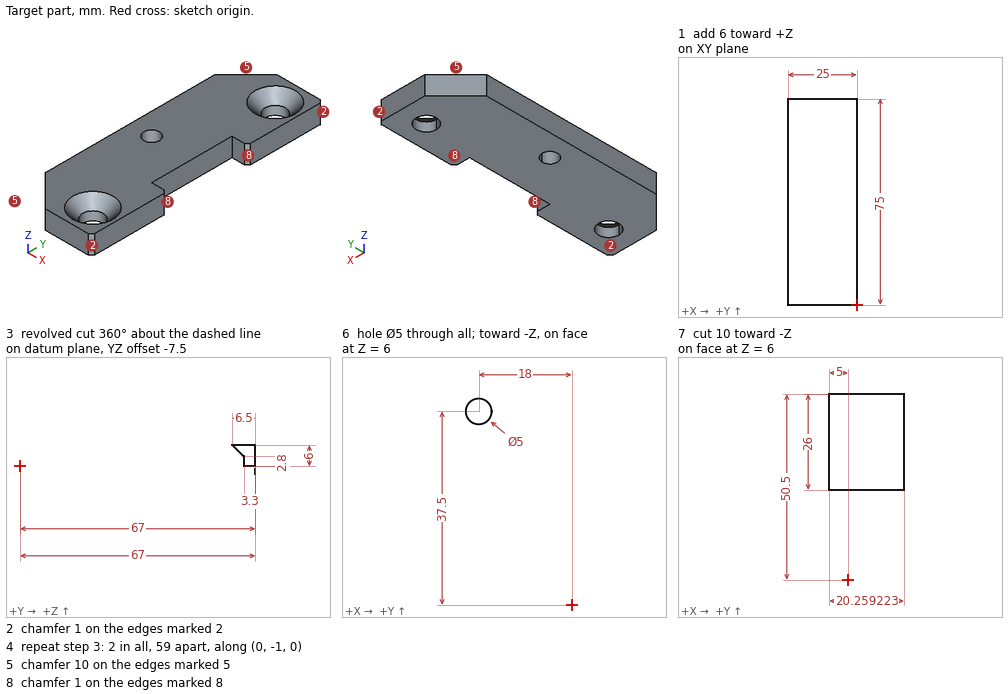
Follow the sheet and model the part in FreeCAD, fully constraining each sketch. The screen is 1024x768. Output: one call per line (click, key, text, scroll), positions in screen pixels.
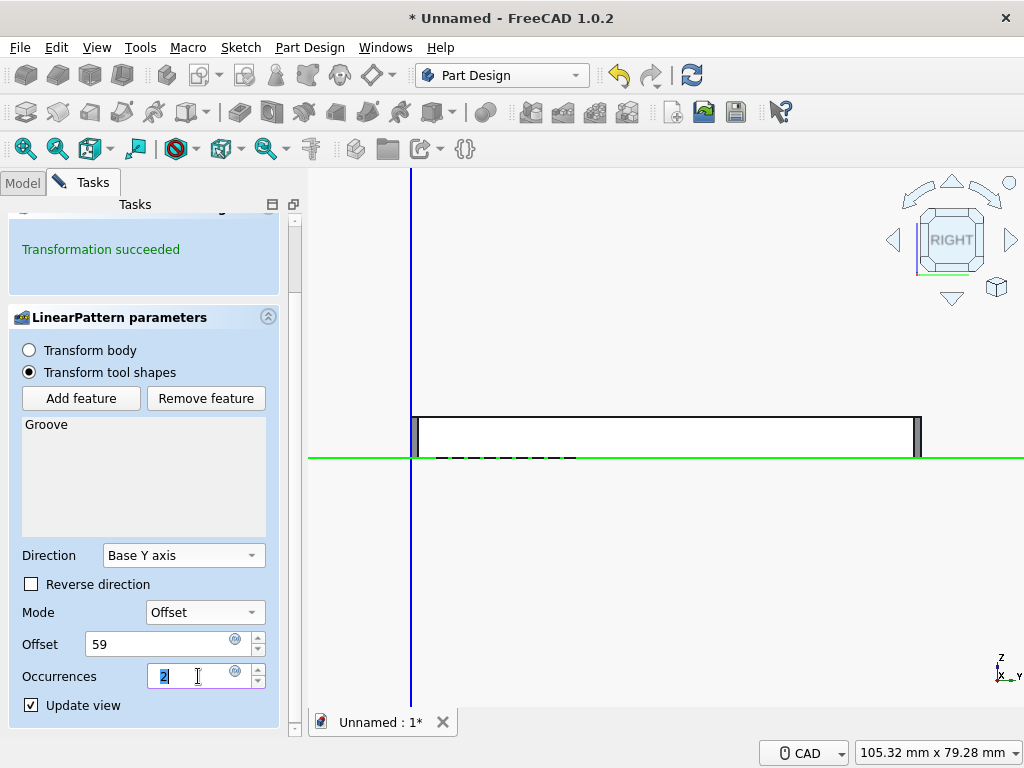
text(2)
key(Tab)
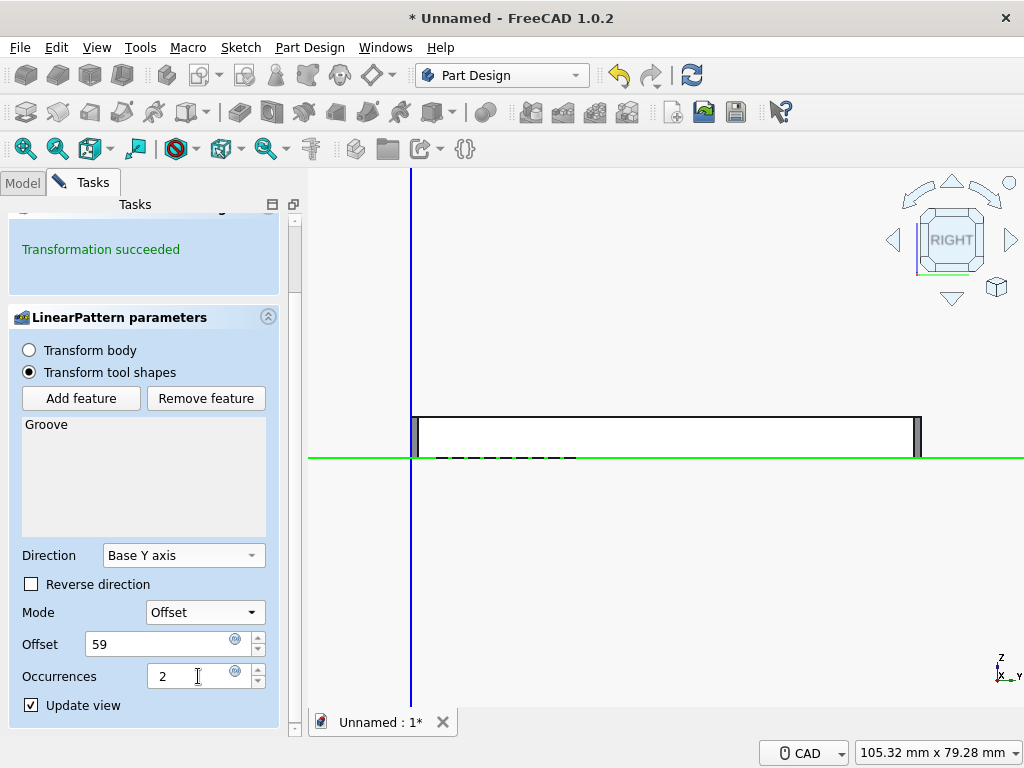
click(30, 584)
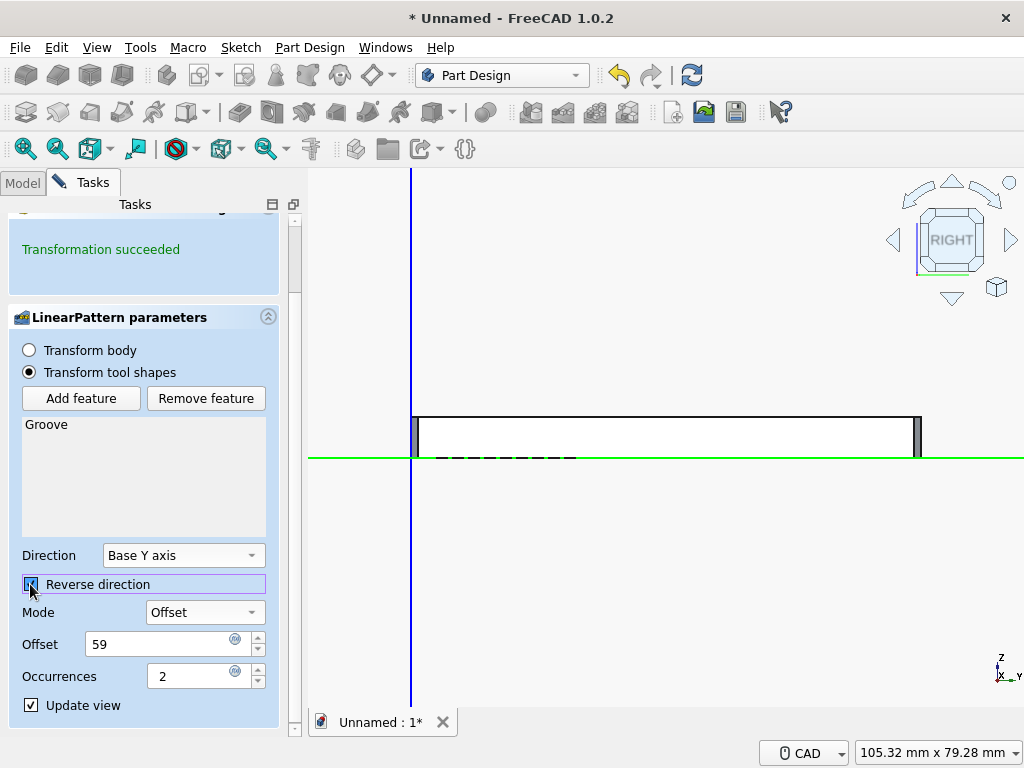
scroll(295, 475, up, 3)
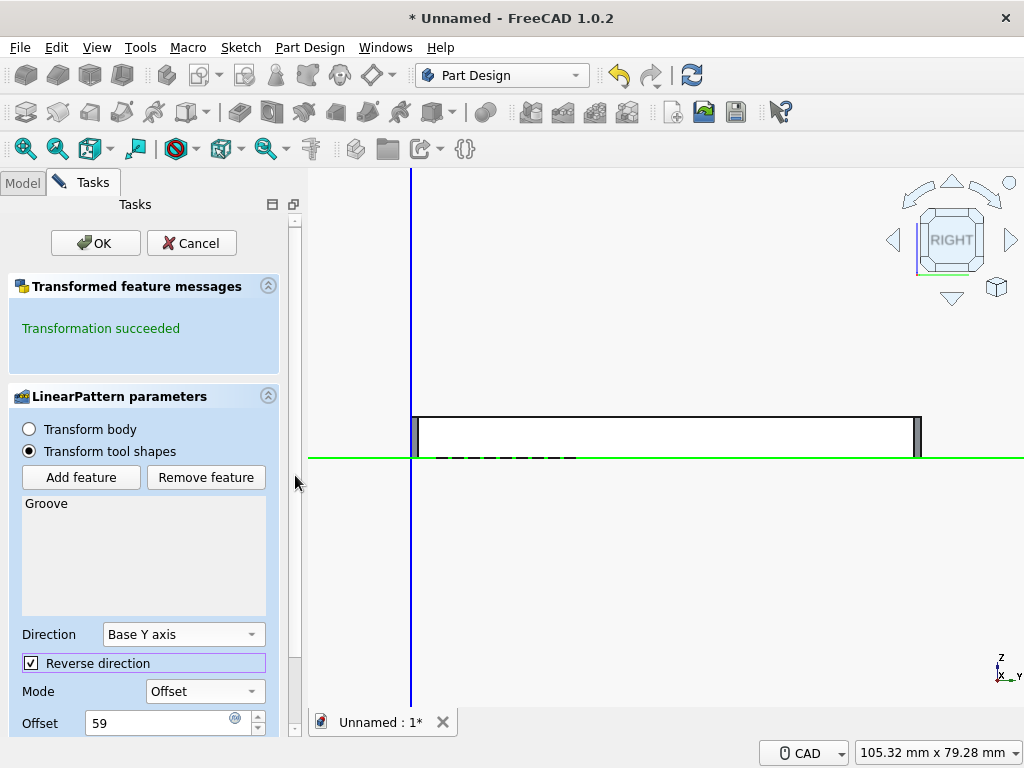
click(96, 243)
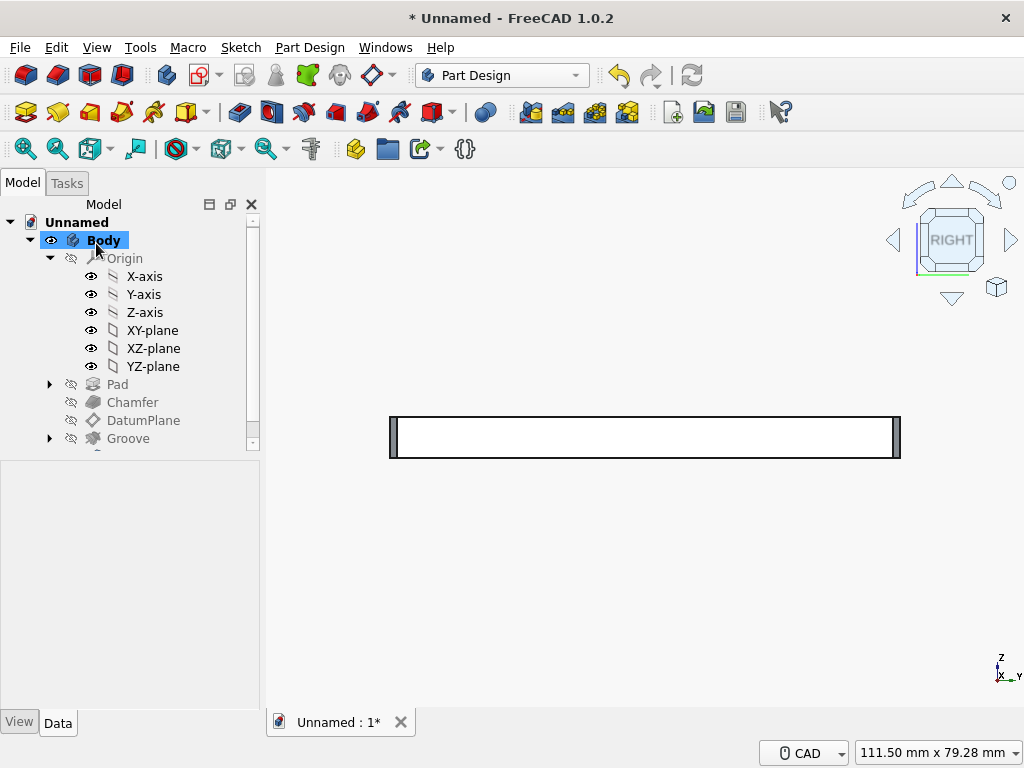
key(0)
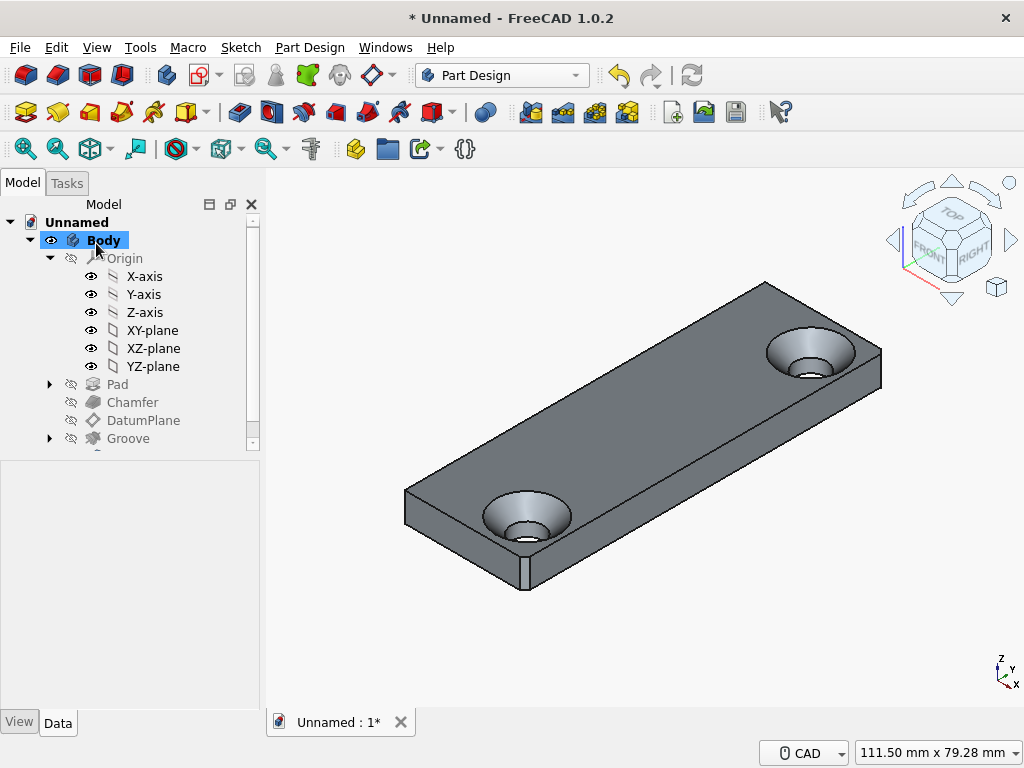
key(2)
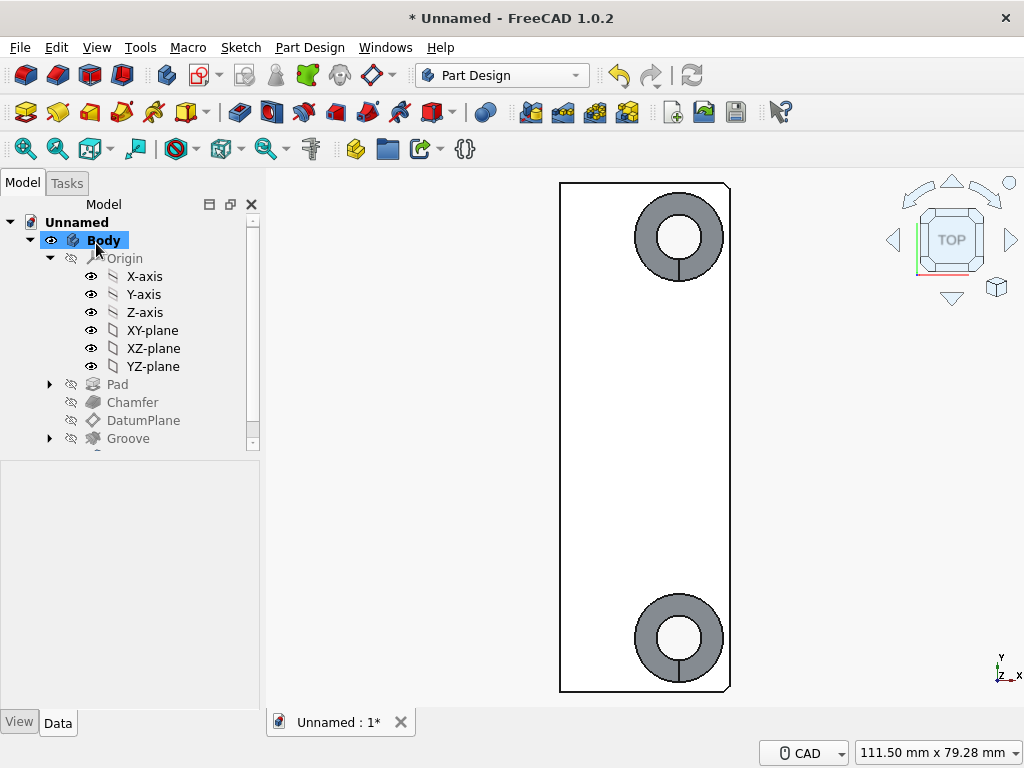
key(1)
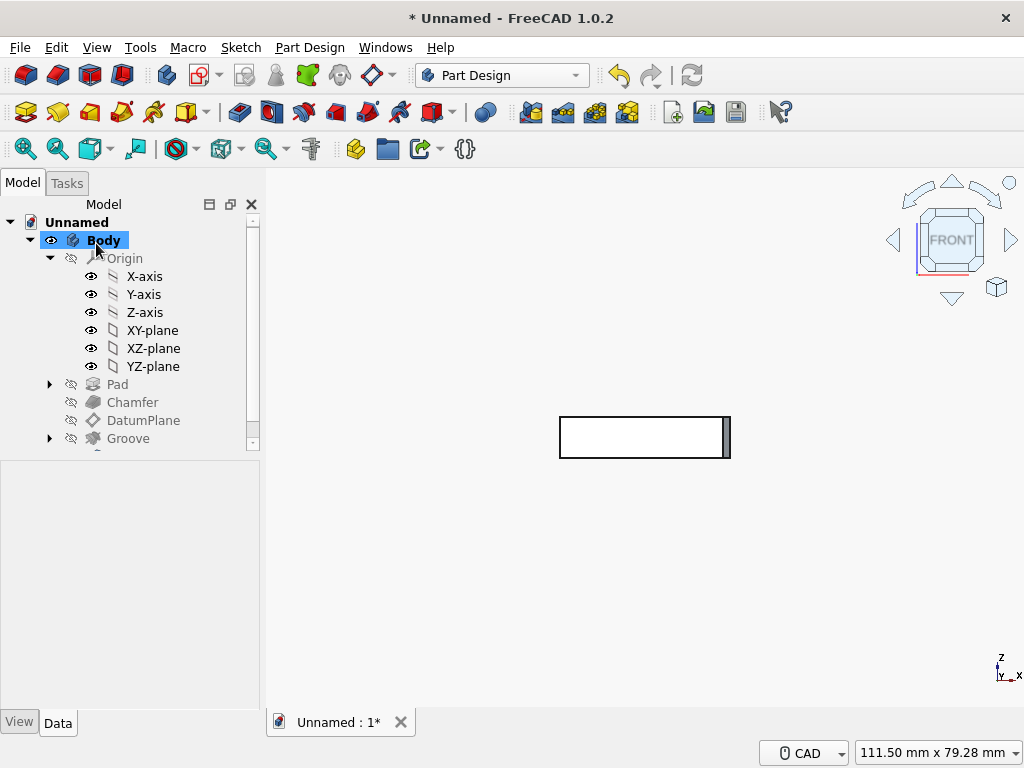
click(26, 150)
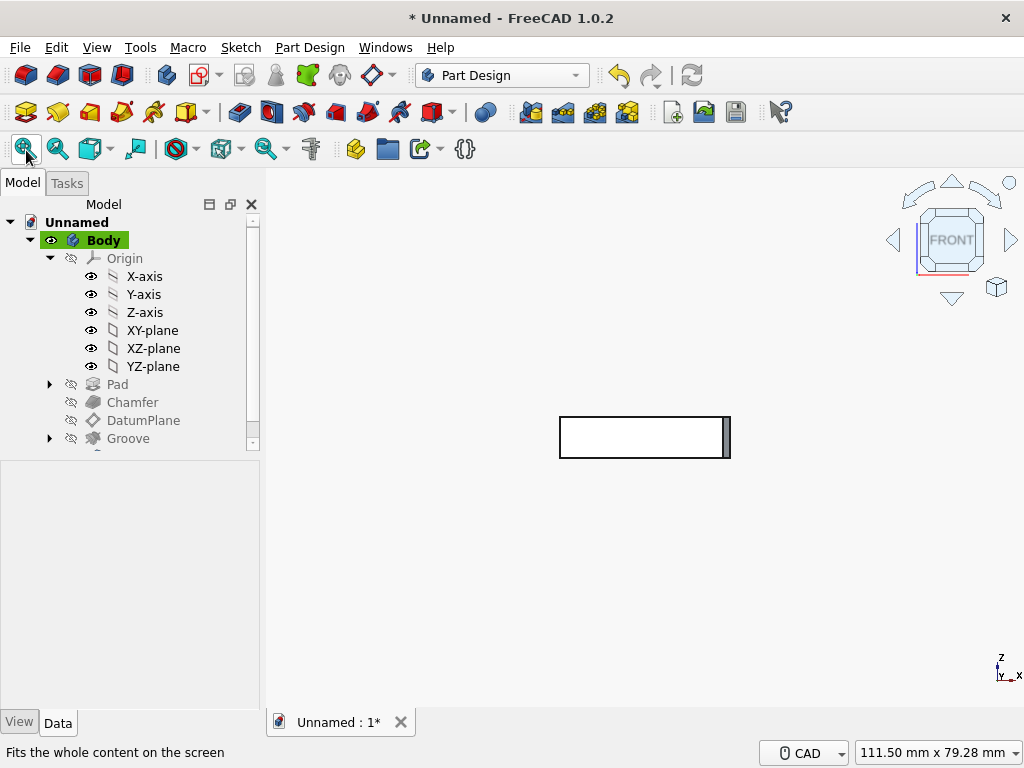
key(3)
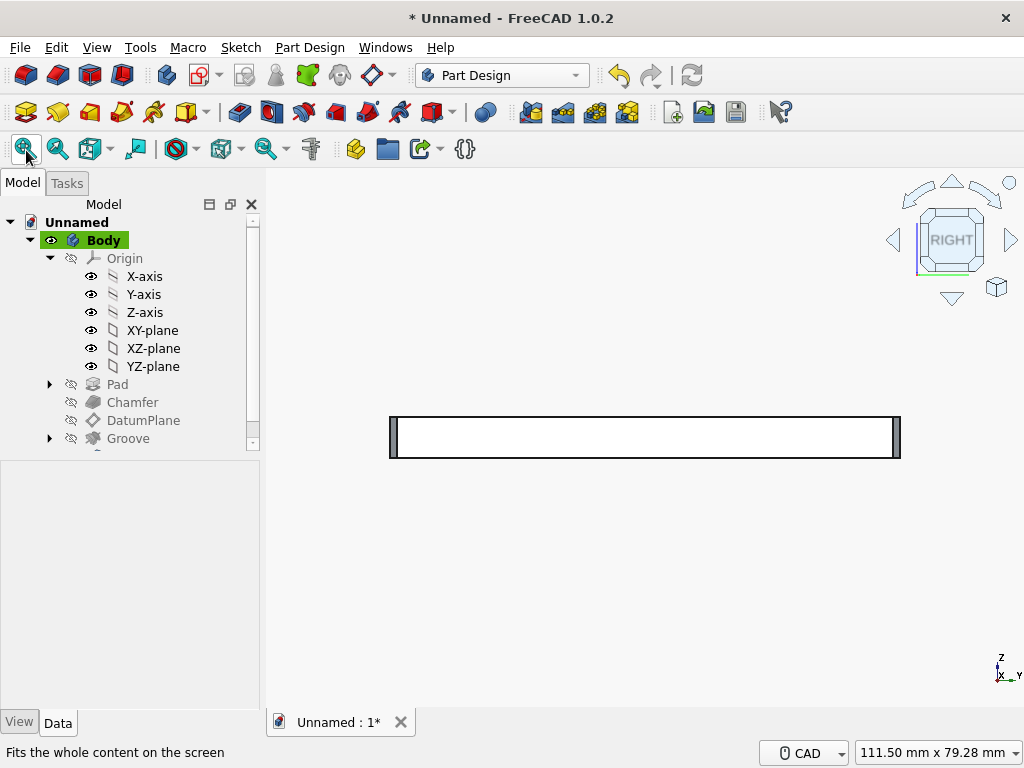
key(5)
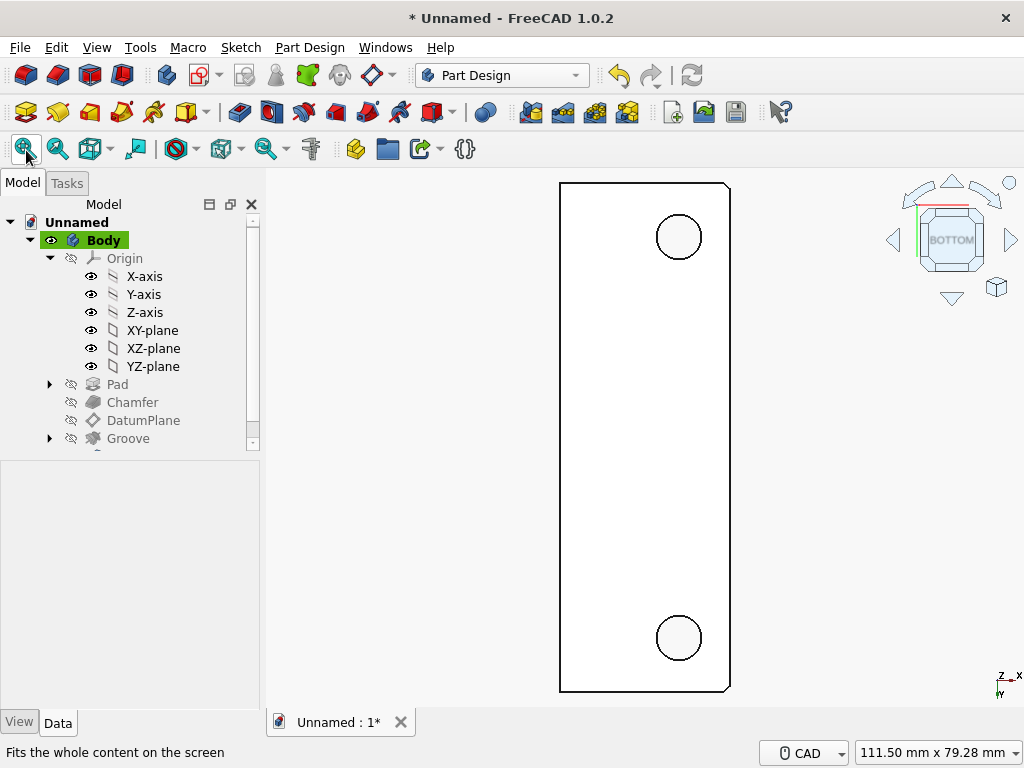
key(4)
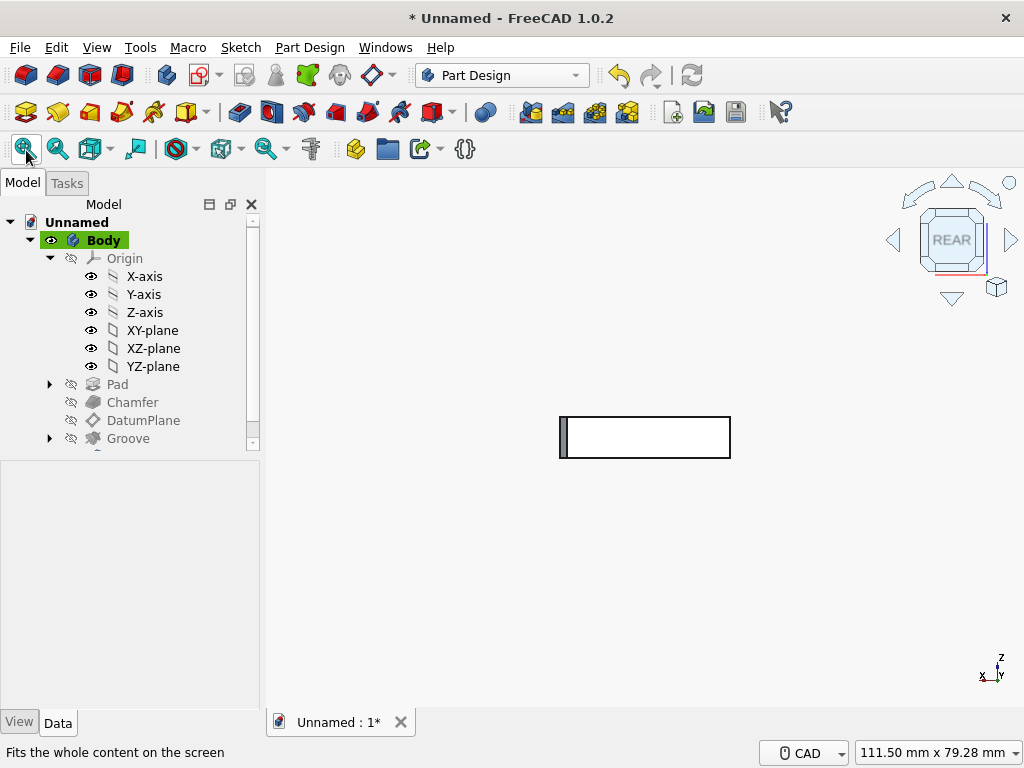
click(26, 150)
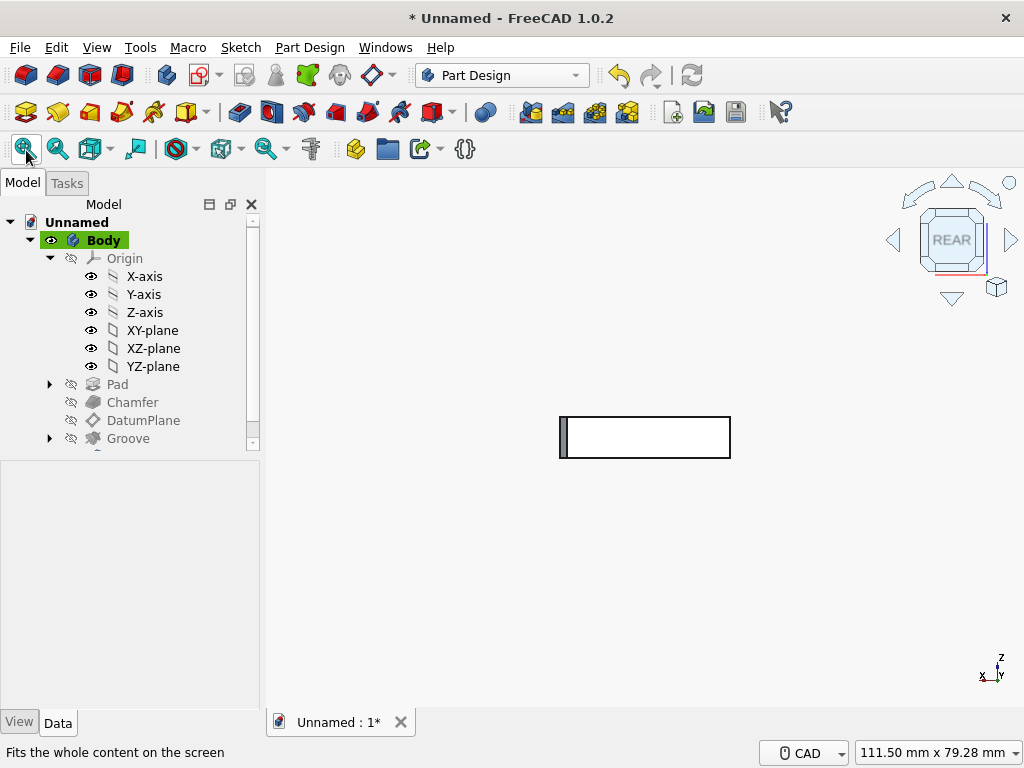
click(730, 437)